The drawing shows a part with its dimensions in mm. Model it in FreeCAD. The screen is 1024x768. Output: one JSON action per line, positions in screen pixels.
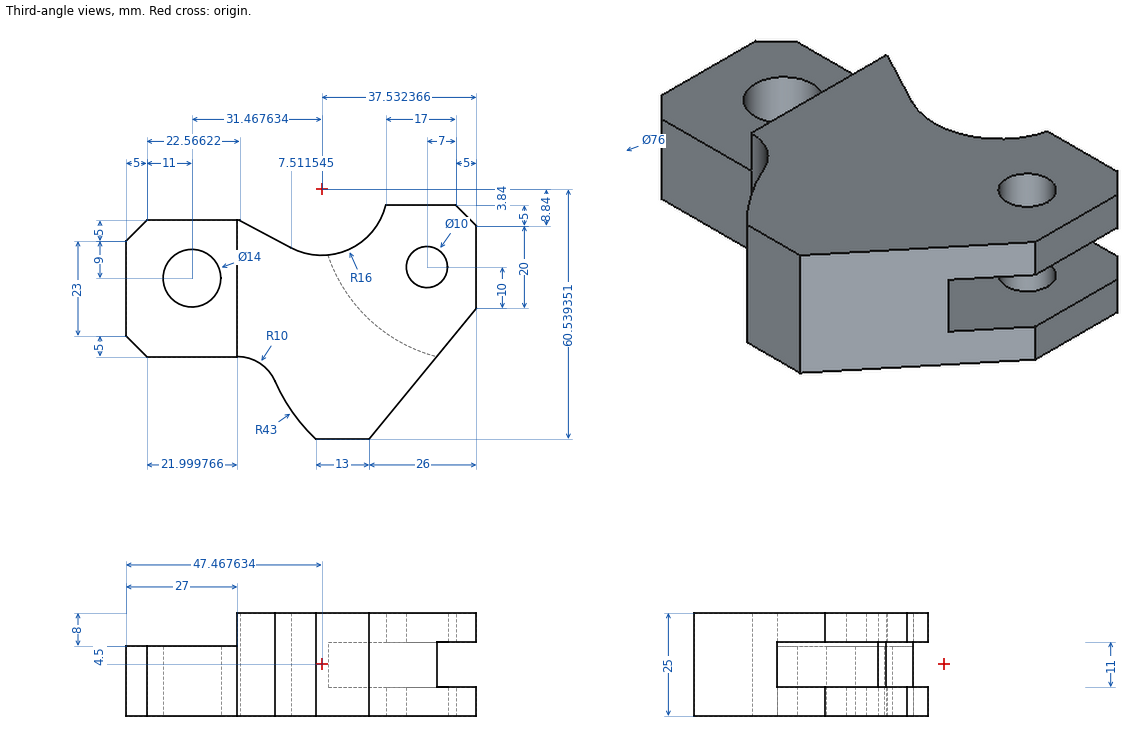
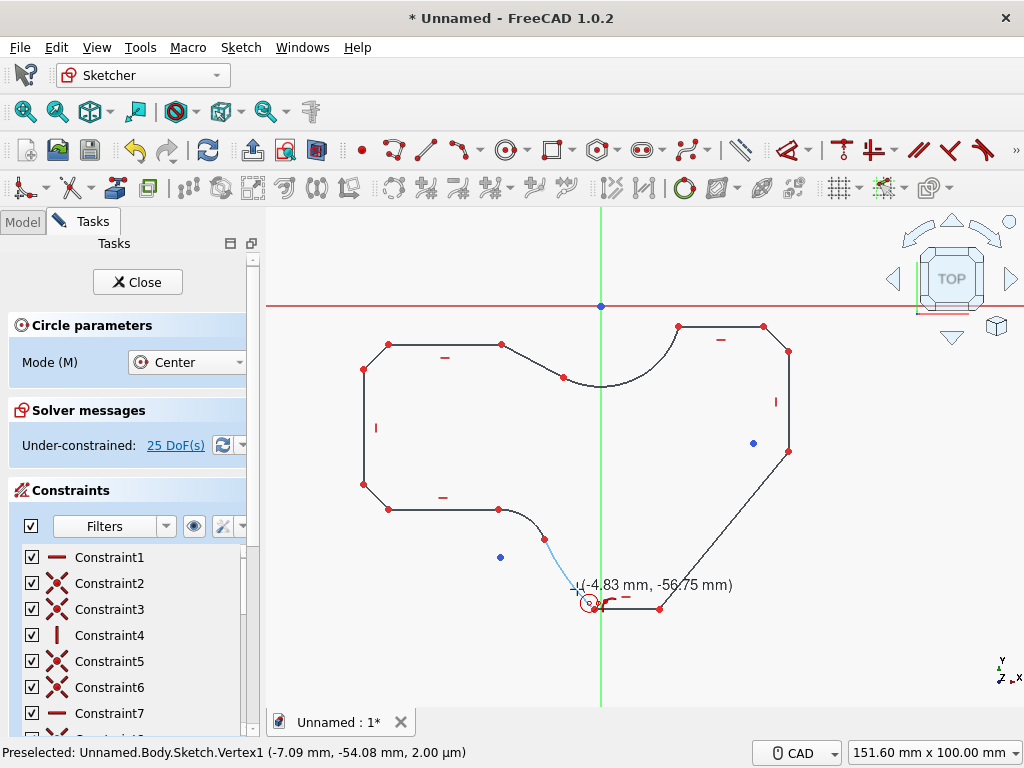
{"action": "left_click", "coordinate": [444, 414]}
{"action": "left_click", "coordinate": [469, 389]}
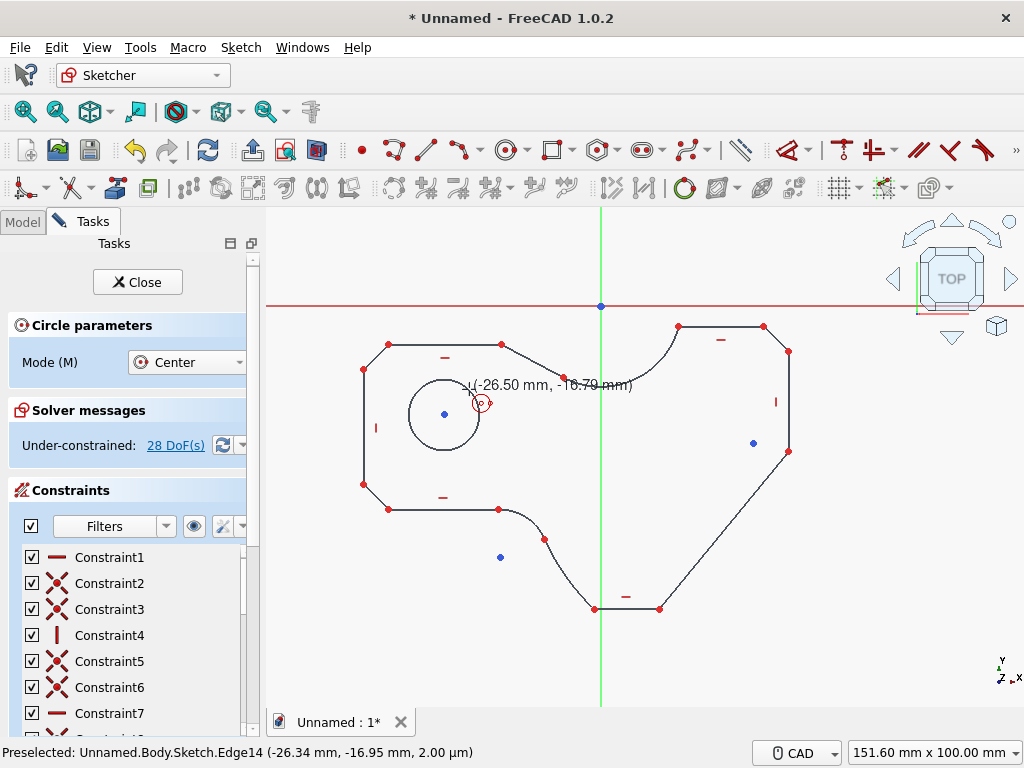
{"action": "left_click", "coordinate": [729, 400]}
{"action": "left_click", "coordinate": [747, 383]}
{"action": "key", "text": "Escape"}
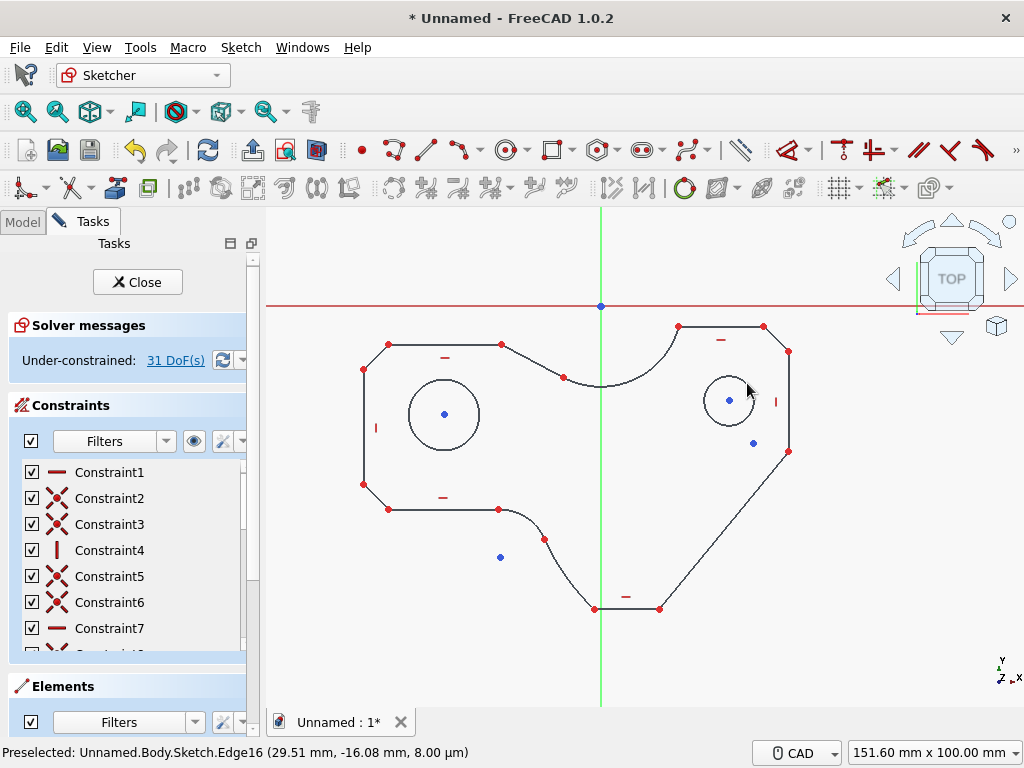
{"action": "left_click", "coordinate": [545, 368]}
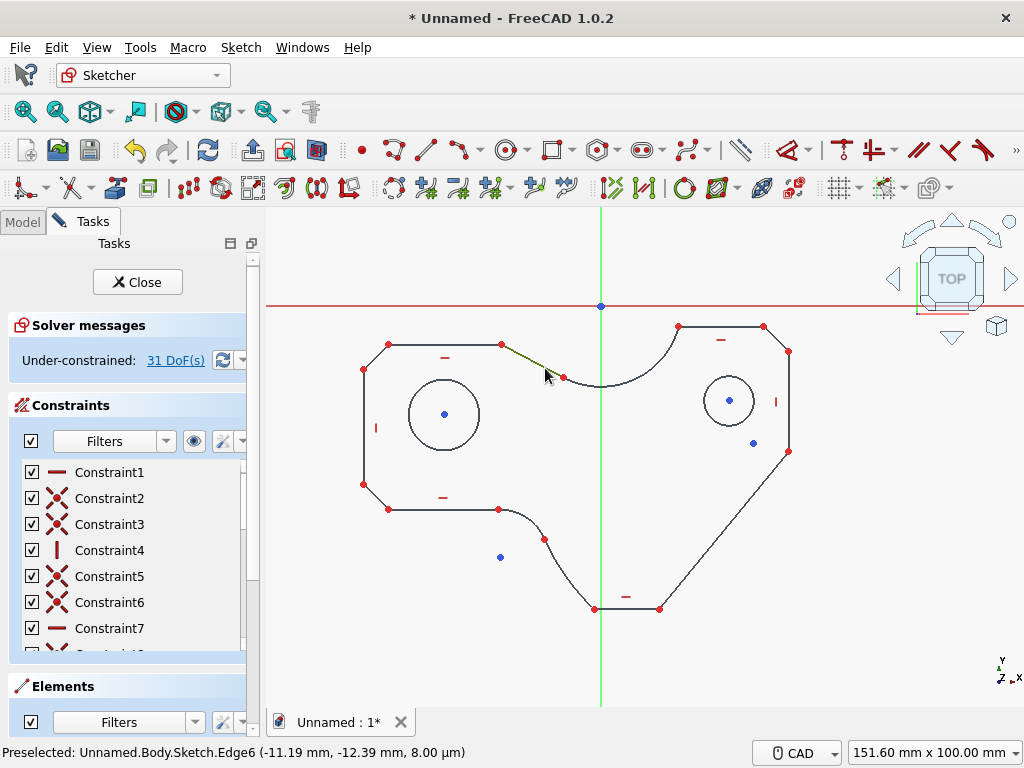
{"action": "left_click", "coordinate": [657, 364]}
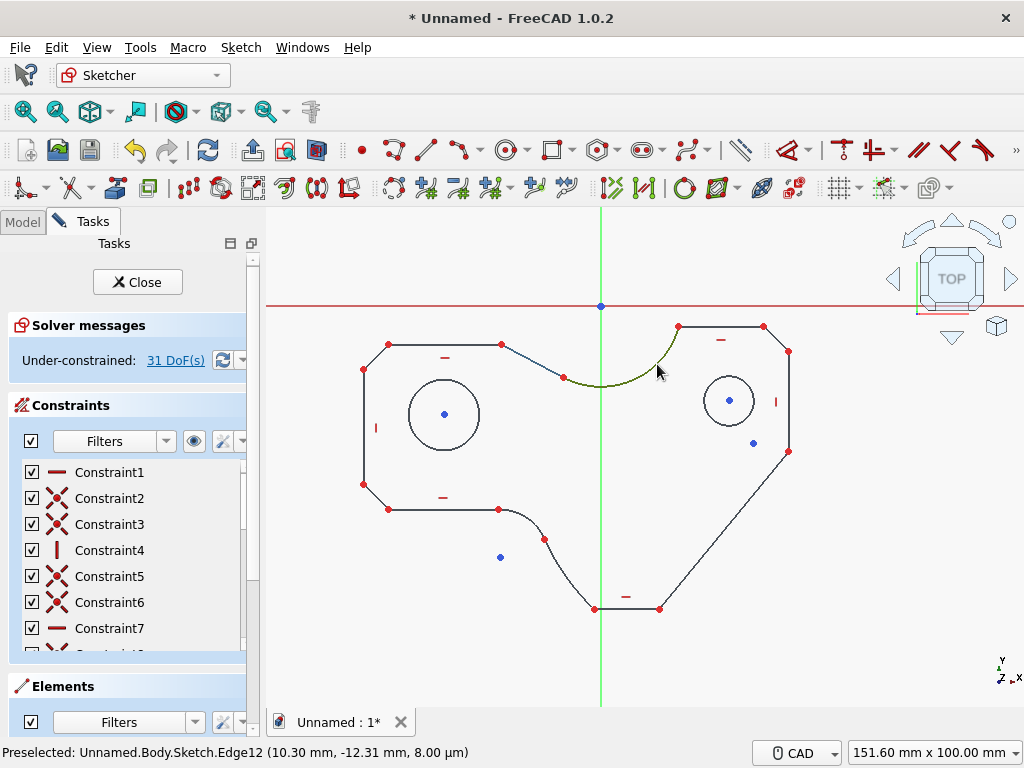
{"action": "left_click", "coordinate": [984, 150]}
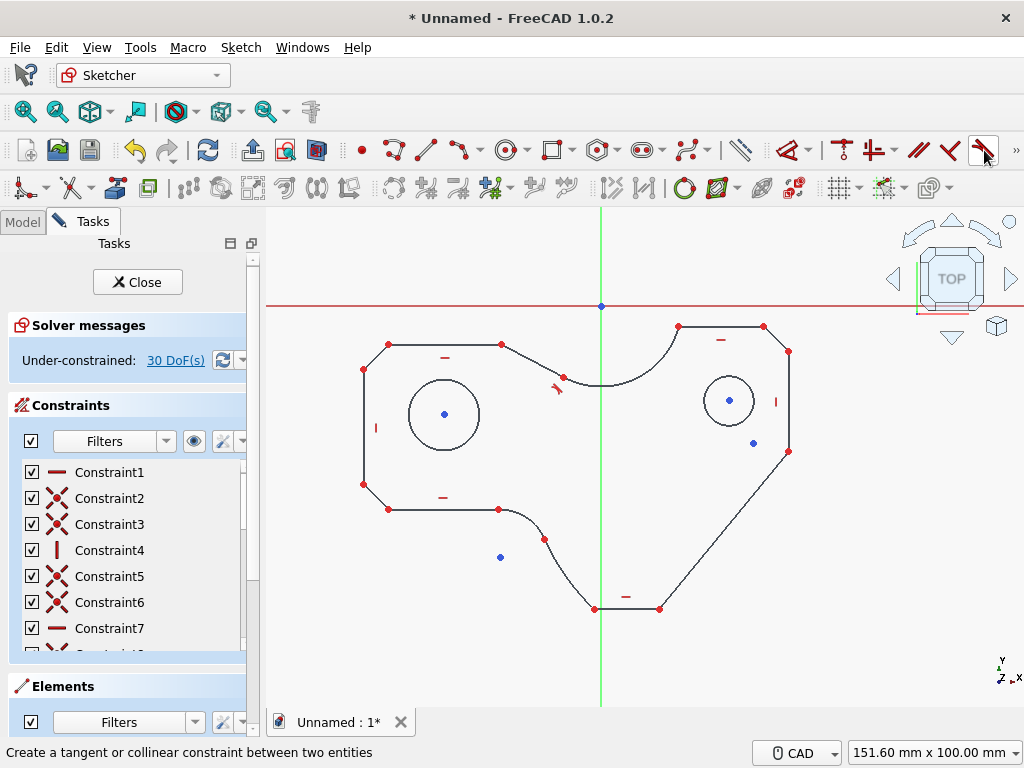
{"action": "left_click", "coordinate": [422, 510]}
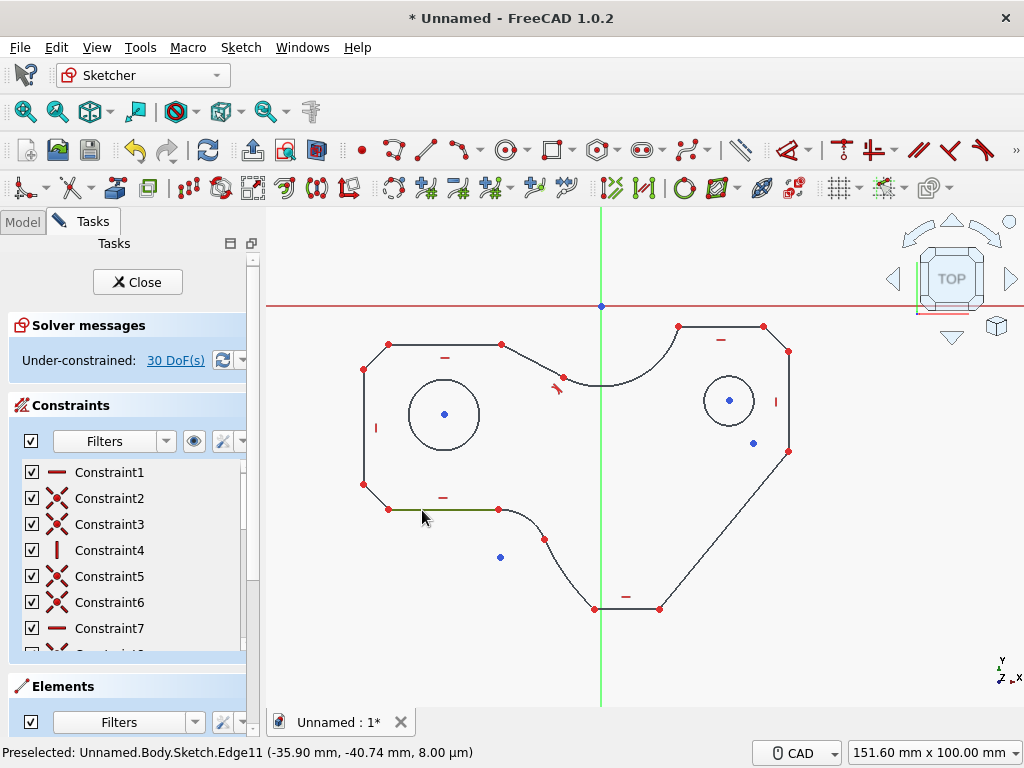
{"action": "left_click", "coordinate": [535, 525]}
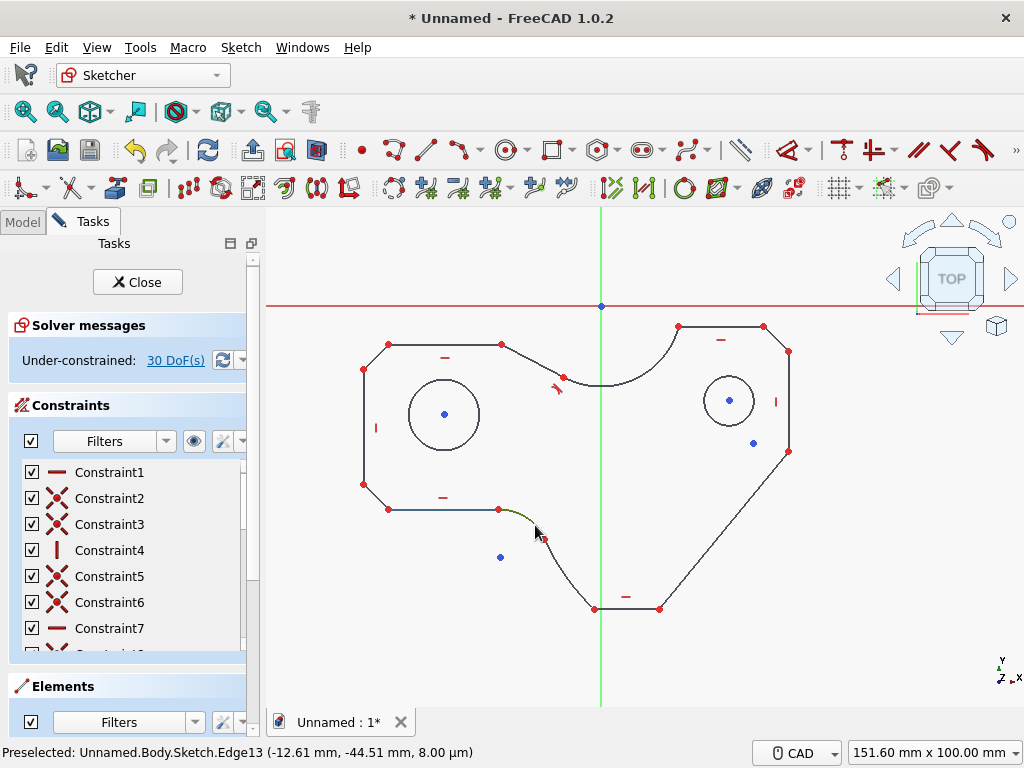
{"action": "left_click", "coordinate": [984, 150]}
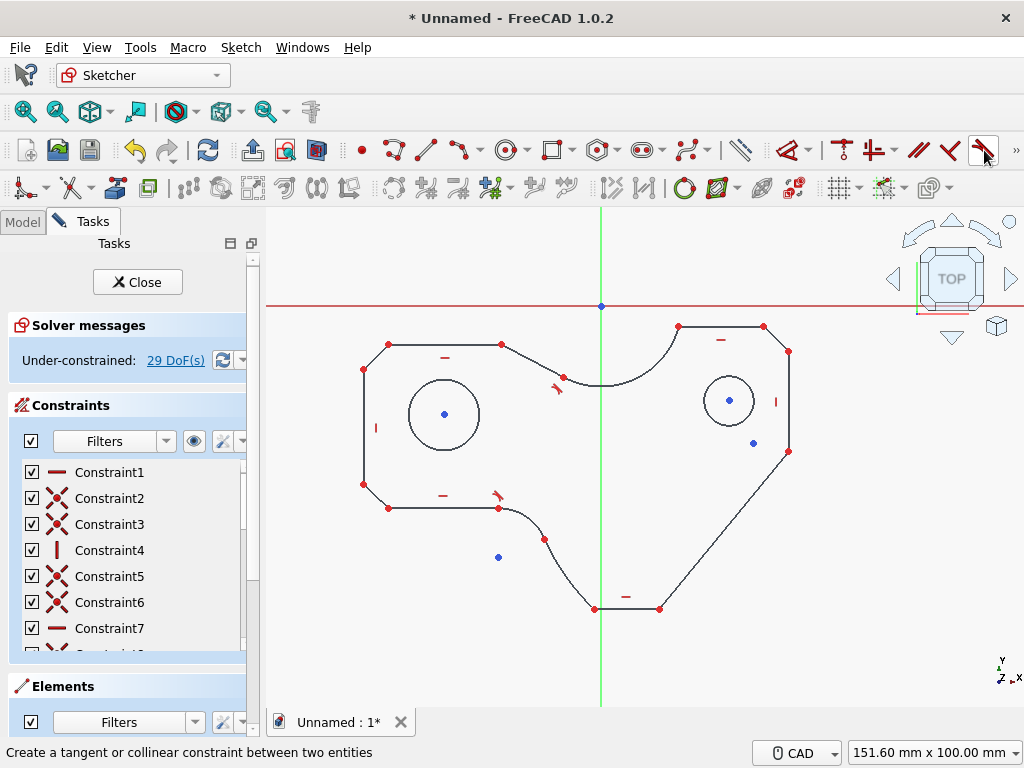
{"action": "left_click", "coordinate": [535, 525]}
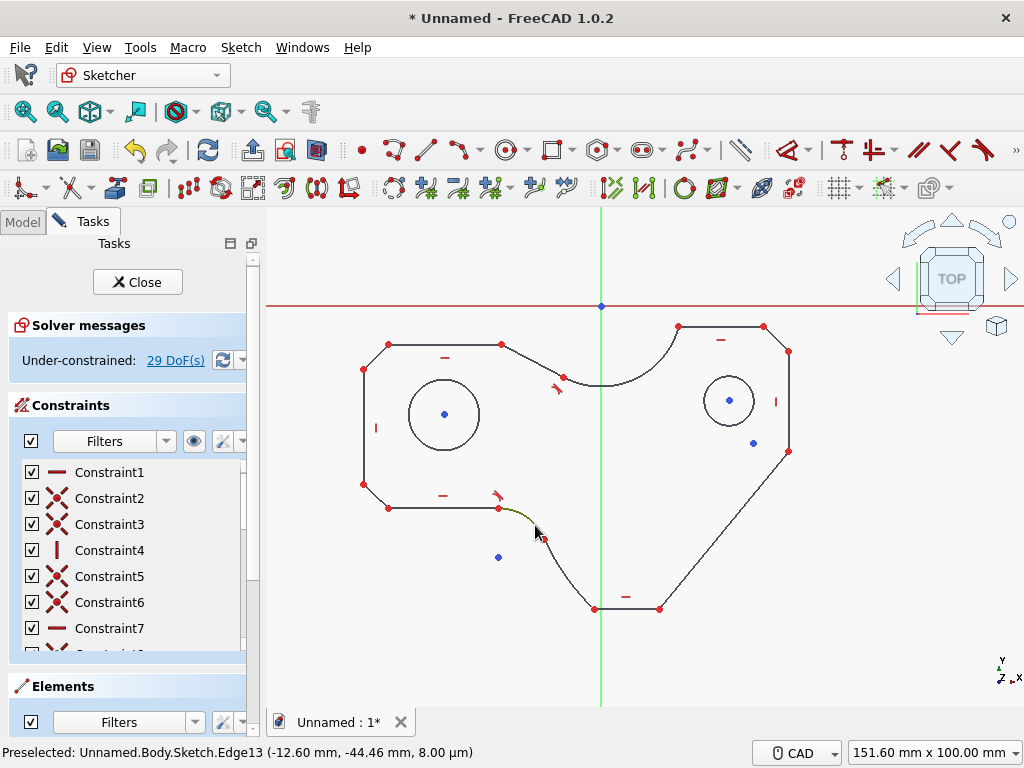
{"action": "left_click", "coordinate": [557, 562]}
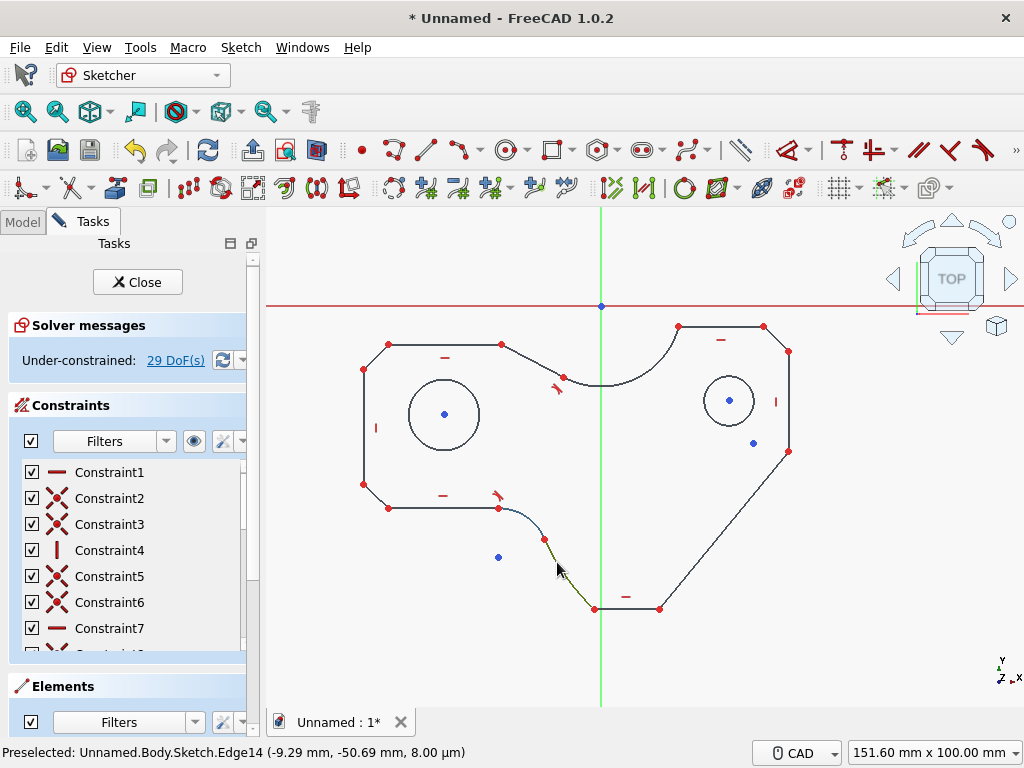
{"action": "left_click", "coordinate": [984, 150]}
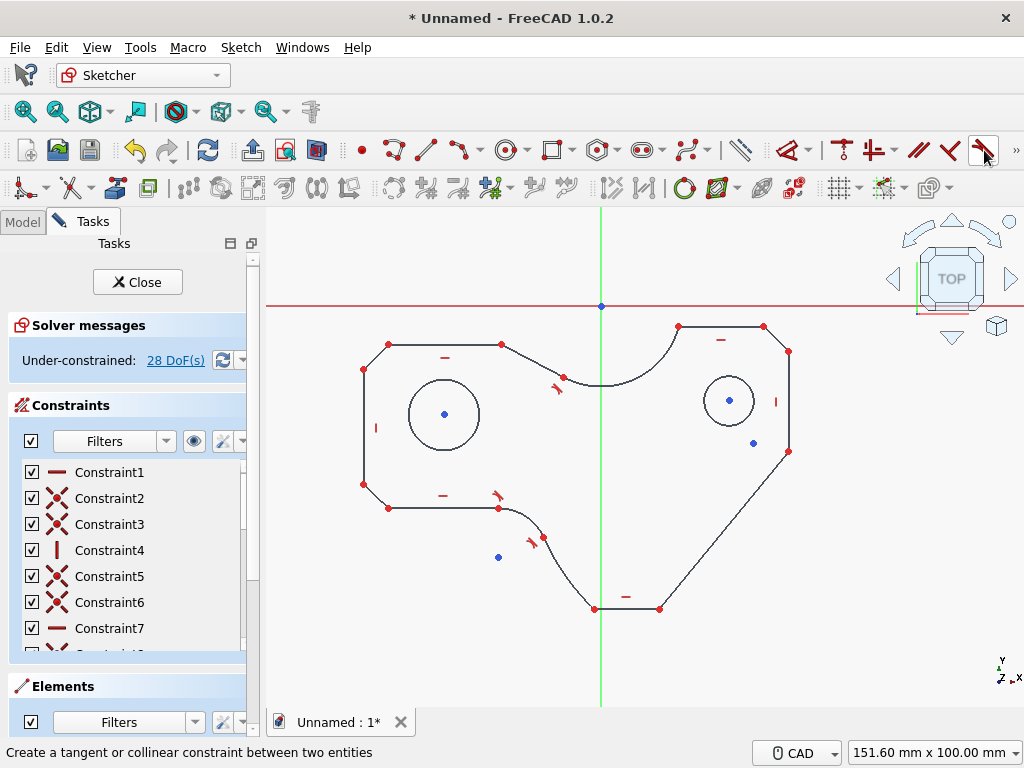
{"action": "scroll", "coordinate": [601, 306], "scroll_direction": "up", "scroll_amount": 3}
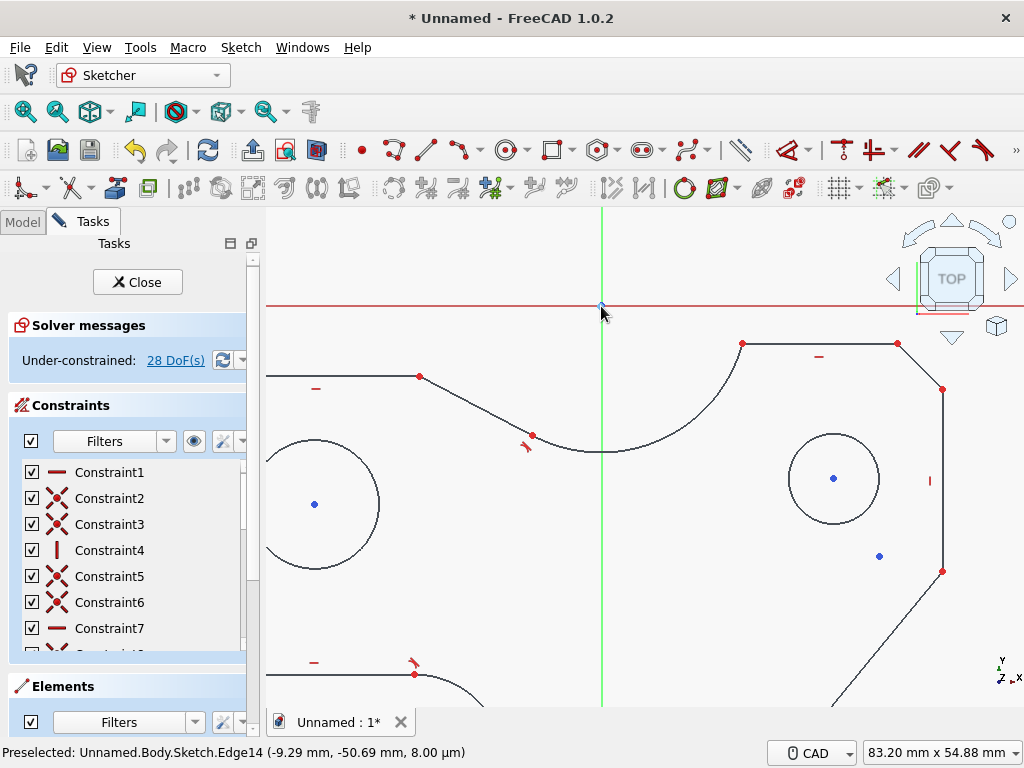
{"action": "left_click_drag", "start_coordinate": [591, 296], "coordinate": [612, 316]}